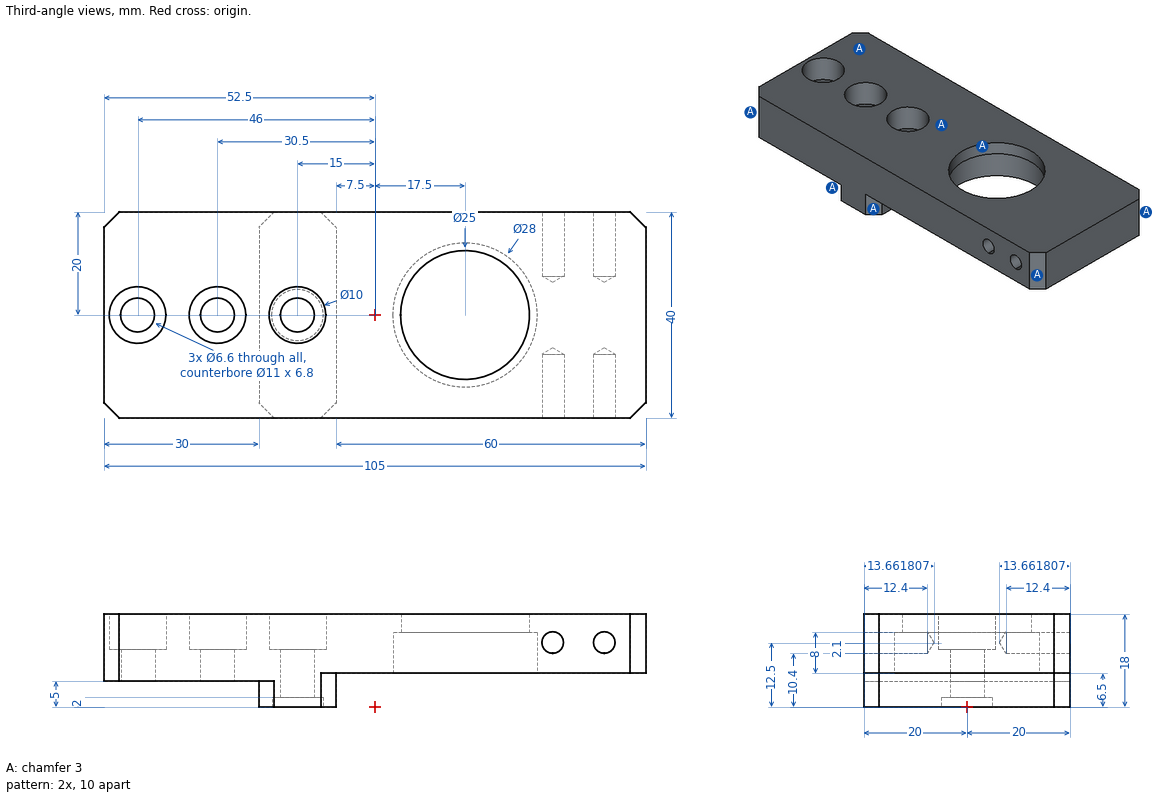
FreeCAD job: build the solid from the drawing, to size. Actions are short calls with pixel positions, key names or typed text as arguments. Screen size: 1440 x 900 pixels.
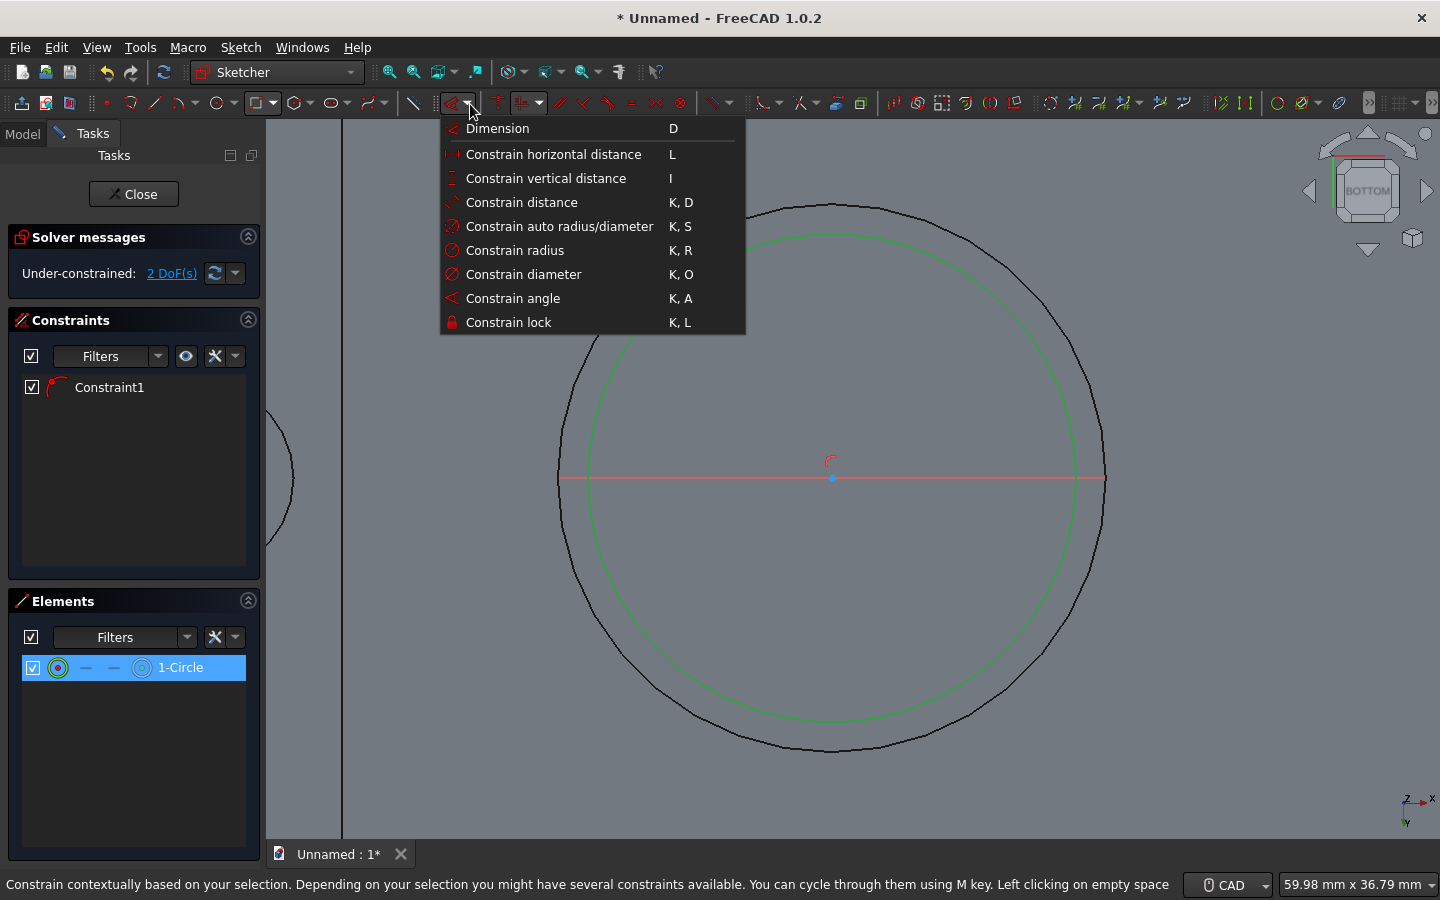
click(593, 274)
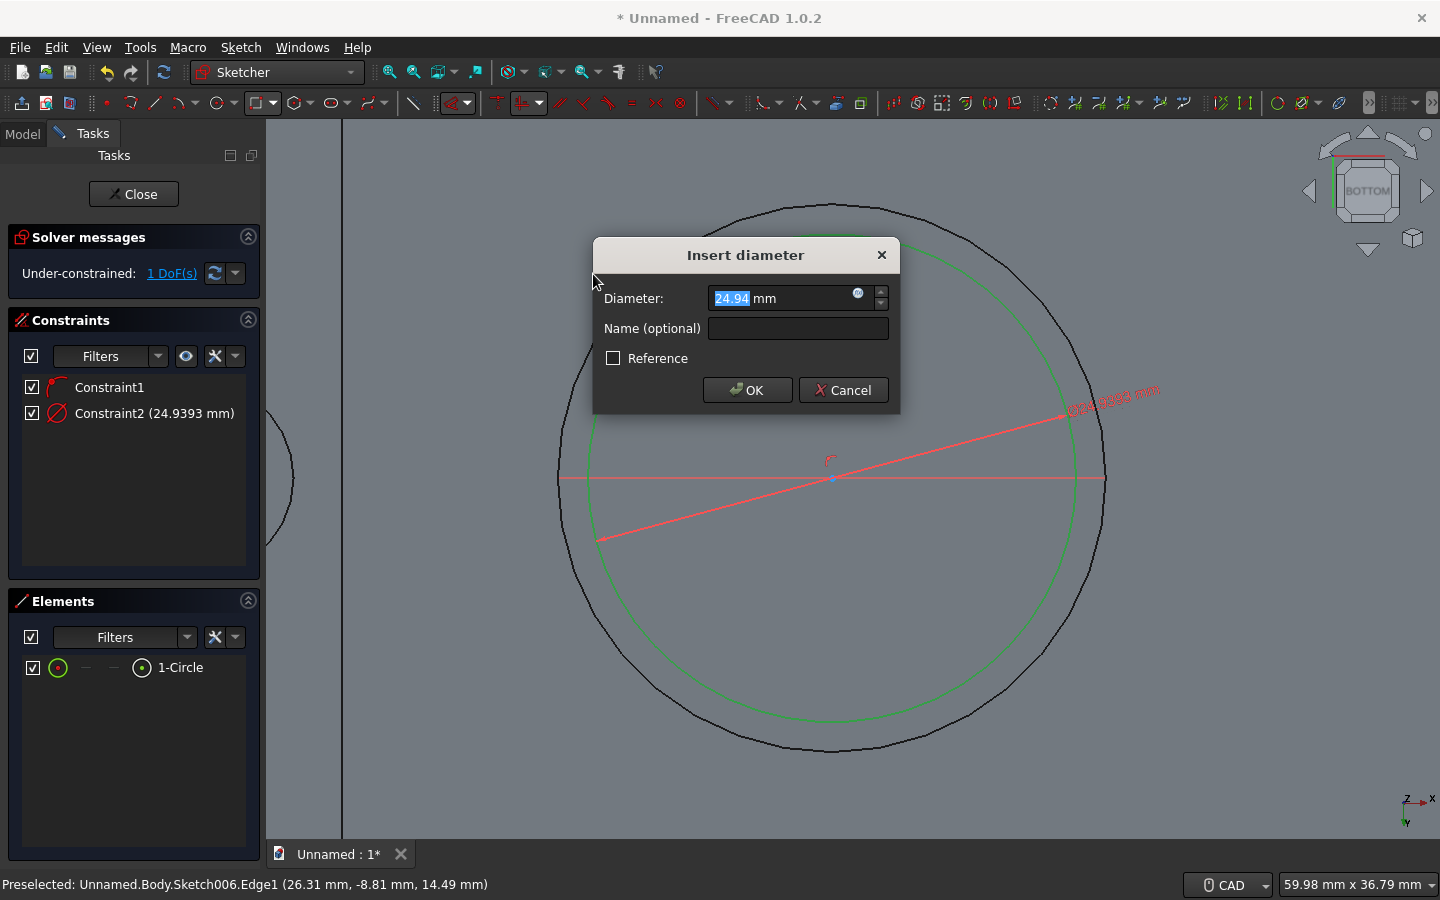
text(25)
key(Return)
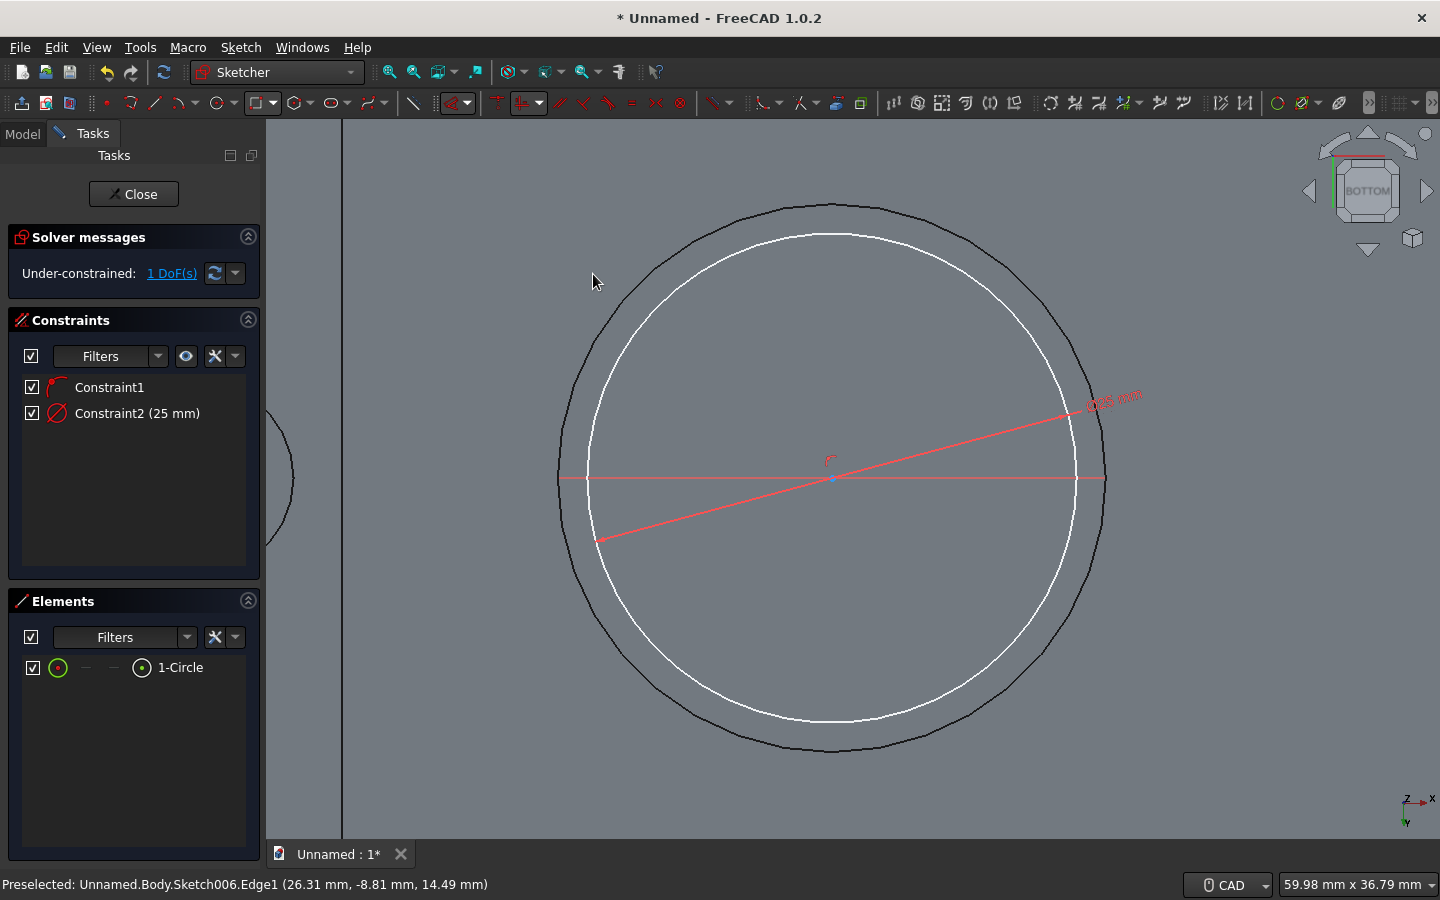
click(832, 478)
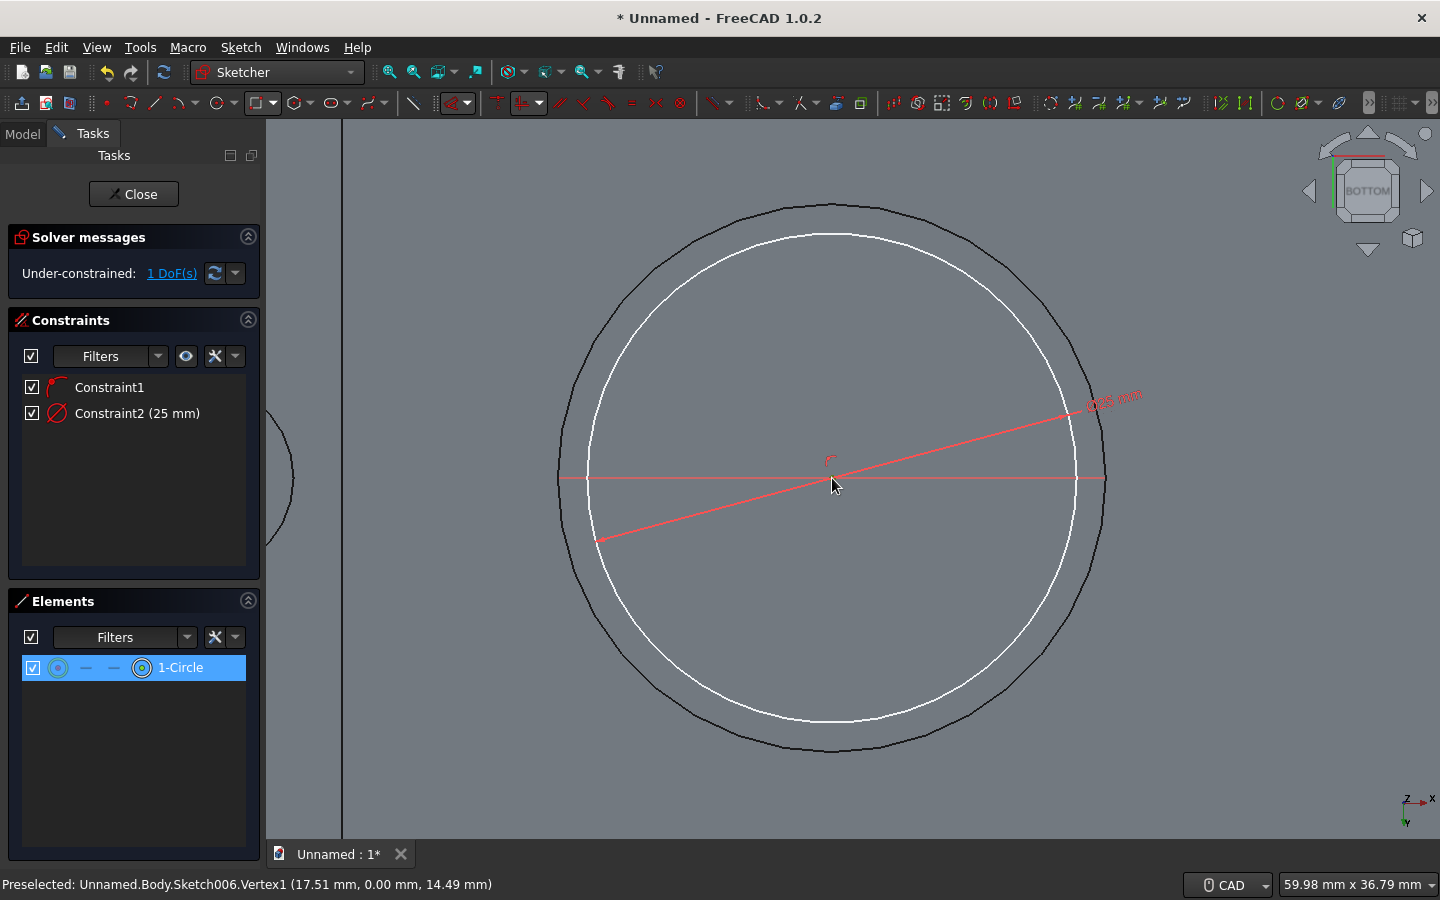
click(470, 104)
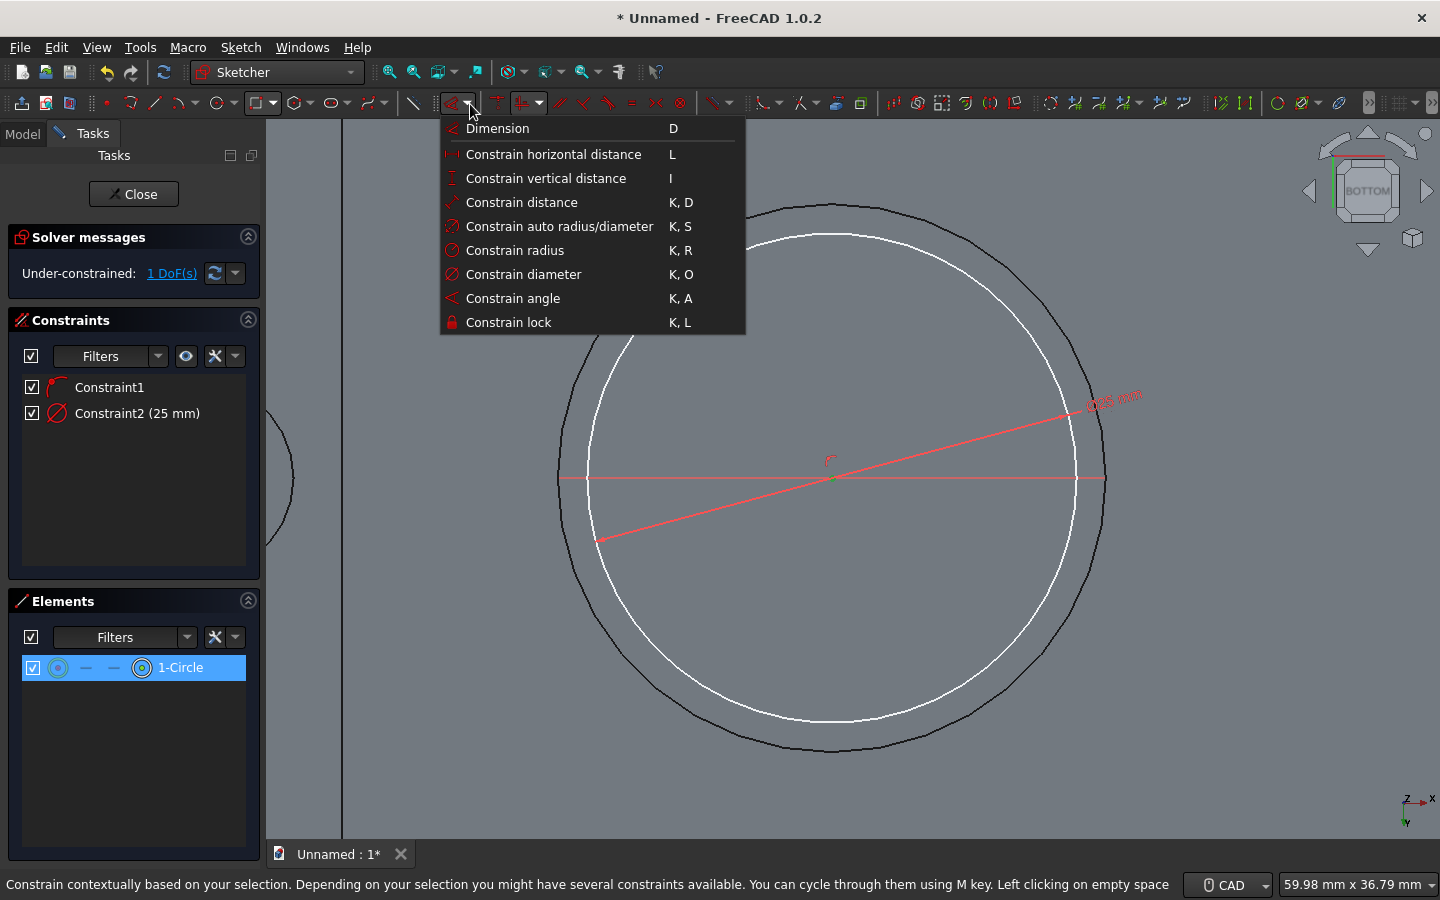
click(593, 154)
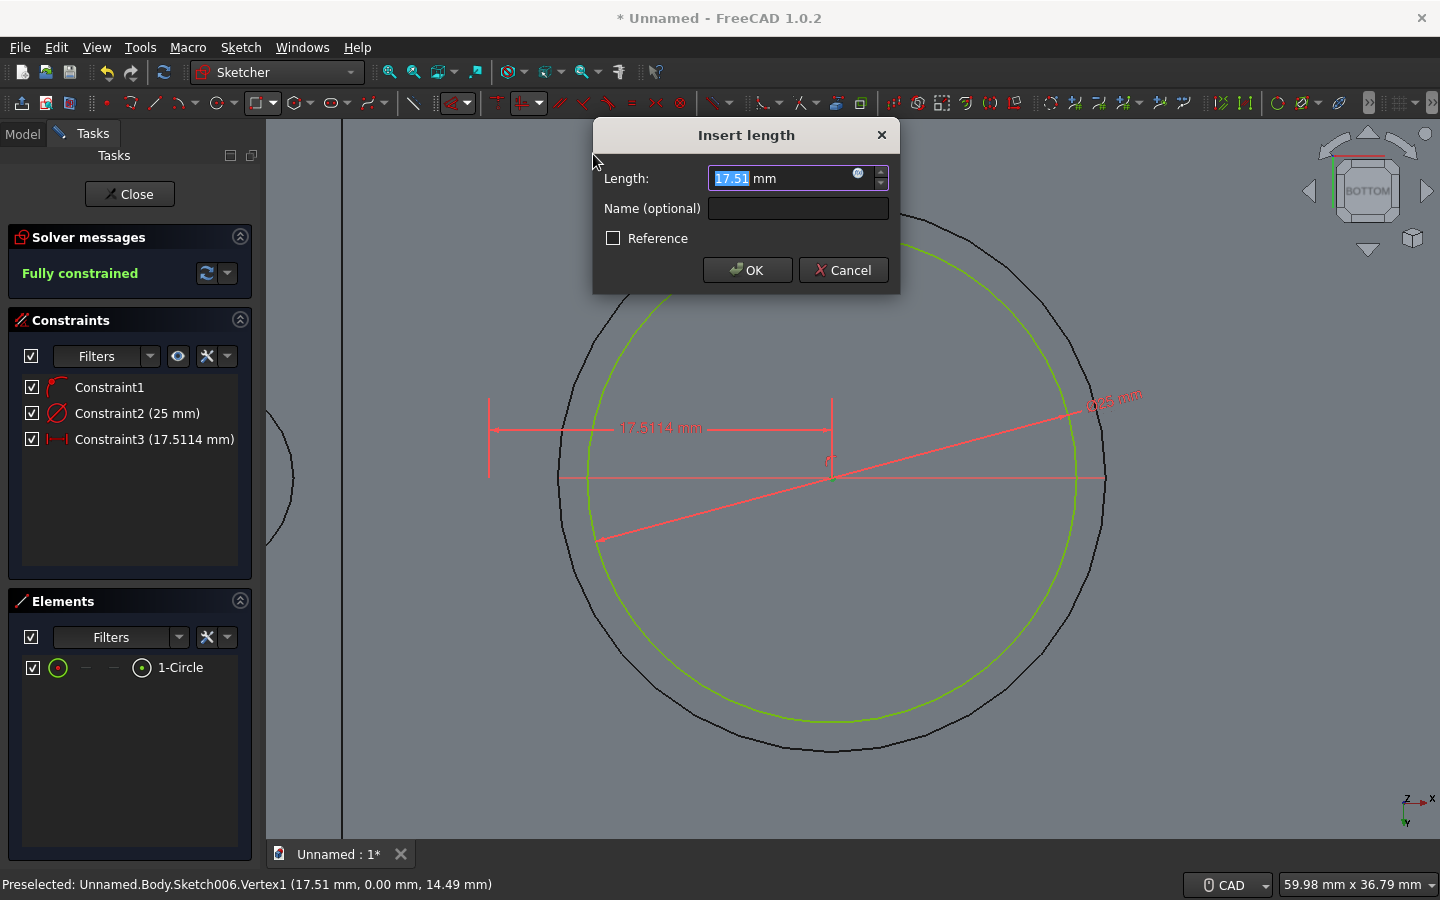
text(17.5)
key(Return)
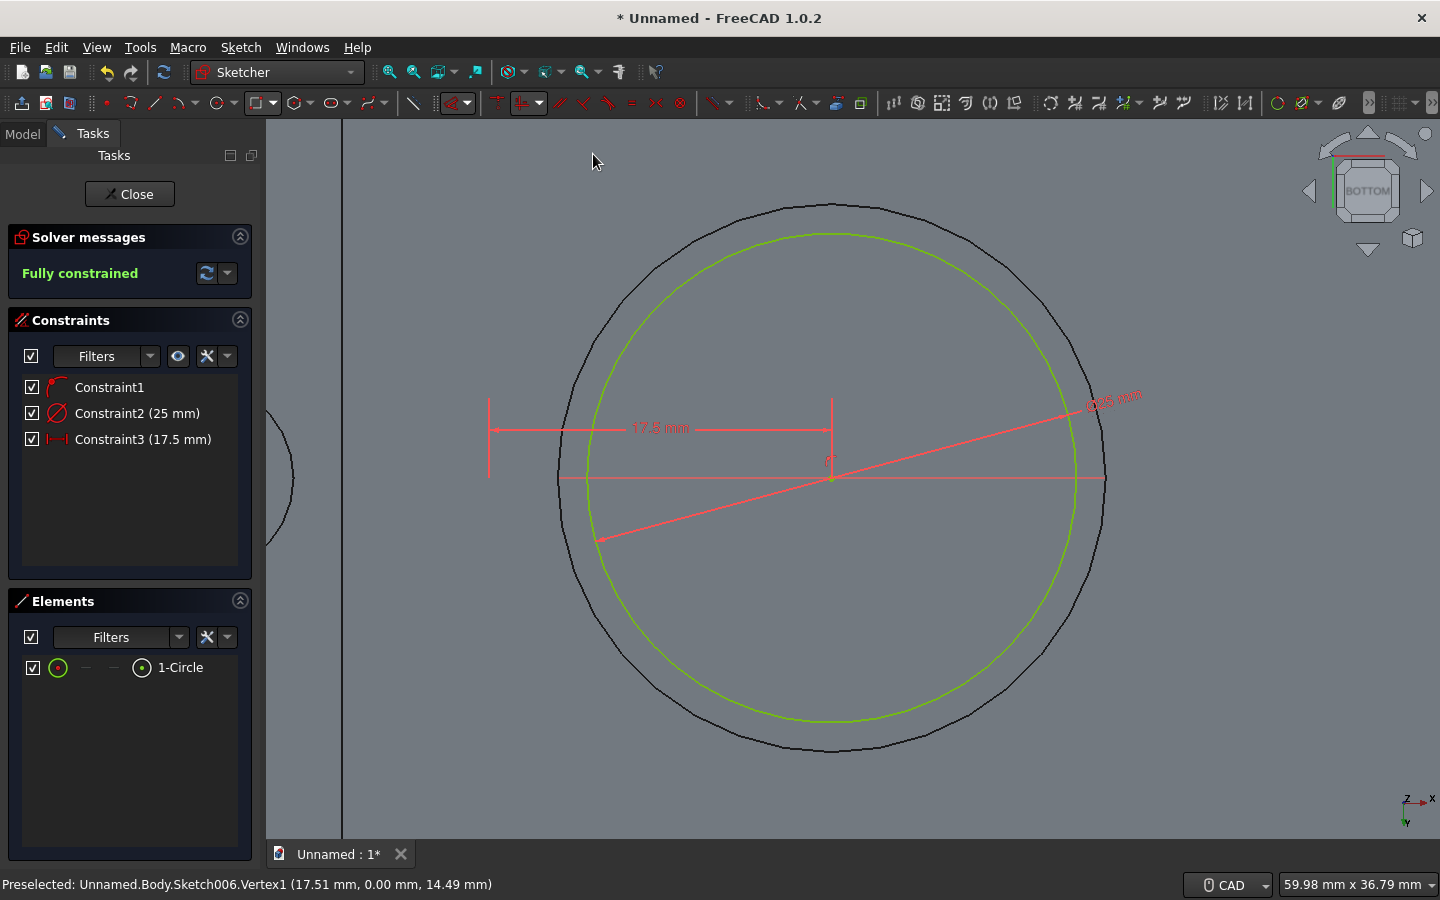
click(130, 194)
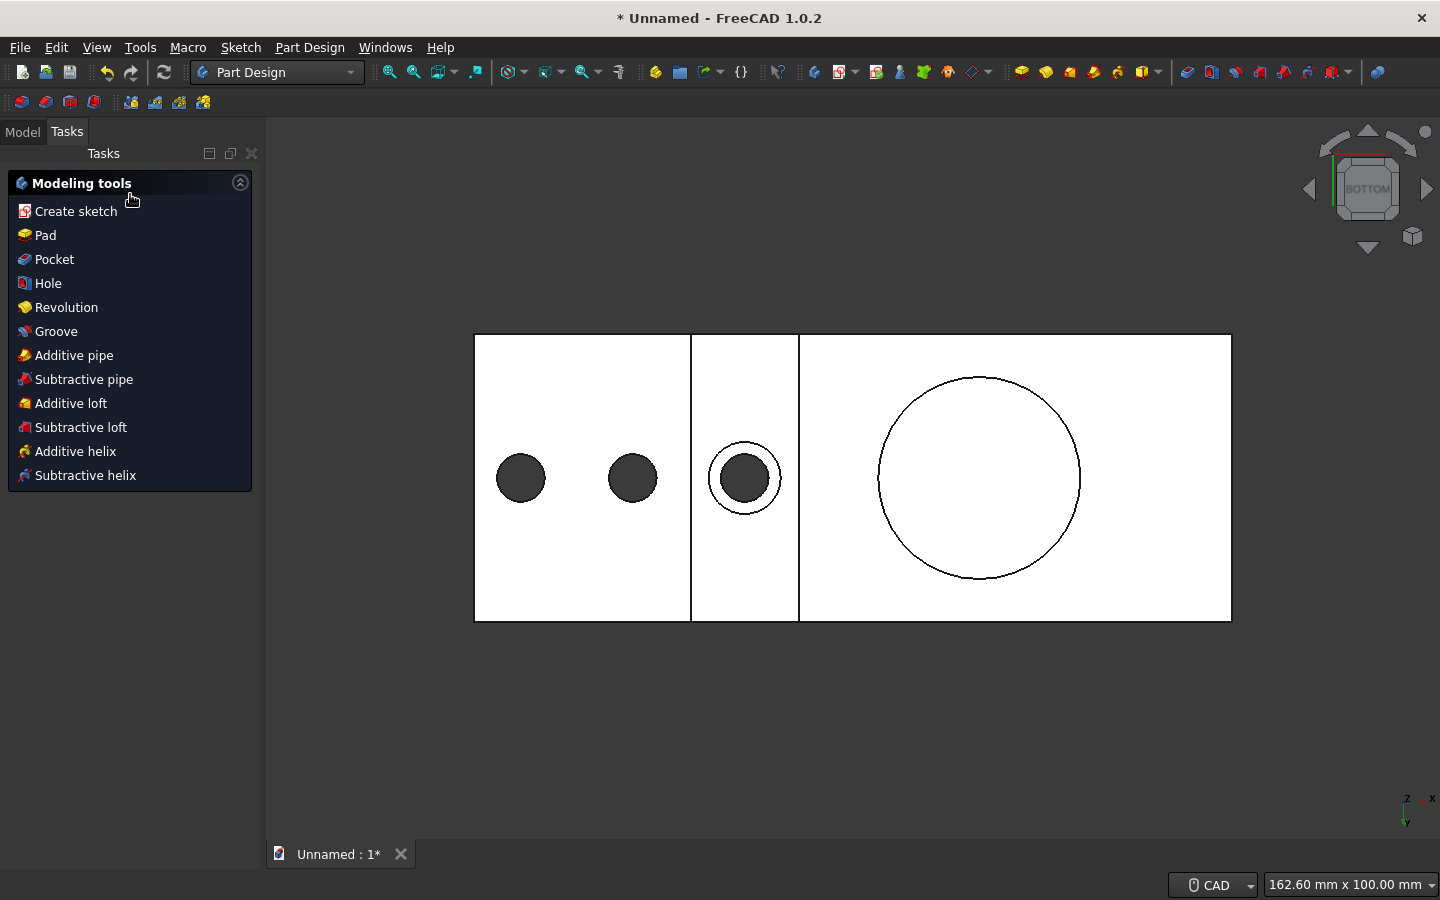
click(1188, 72)